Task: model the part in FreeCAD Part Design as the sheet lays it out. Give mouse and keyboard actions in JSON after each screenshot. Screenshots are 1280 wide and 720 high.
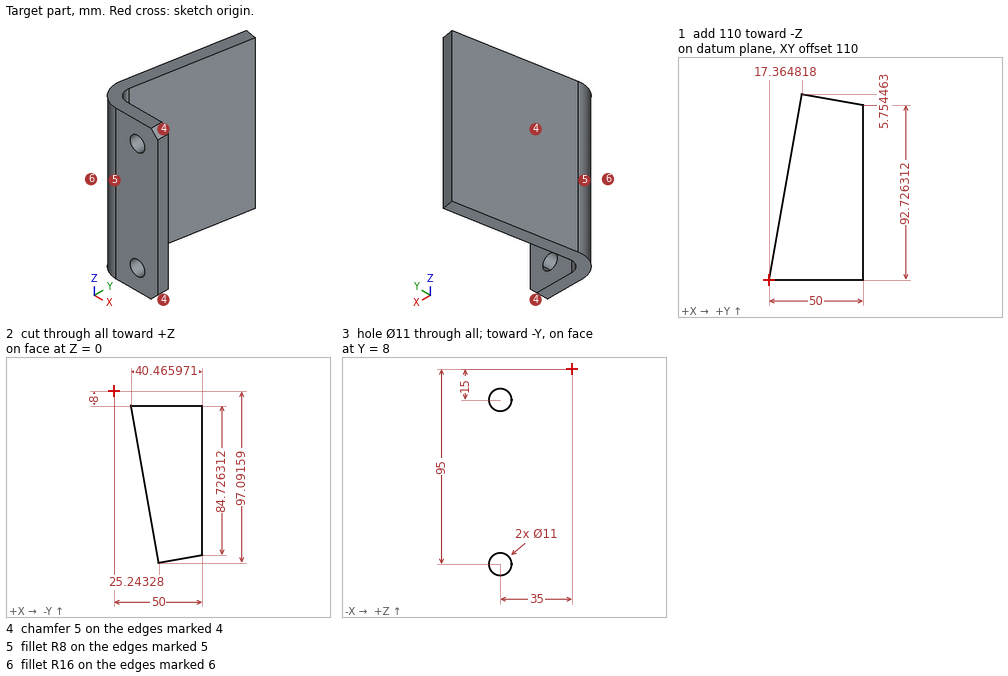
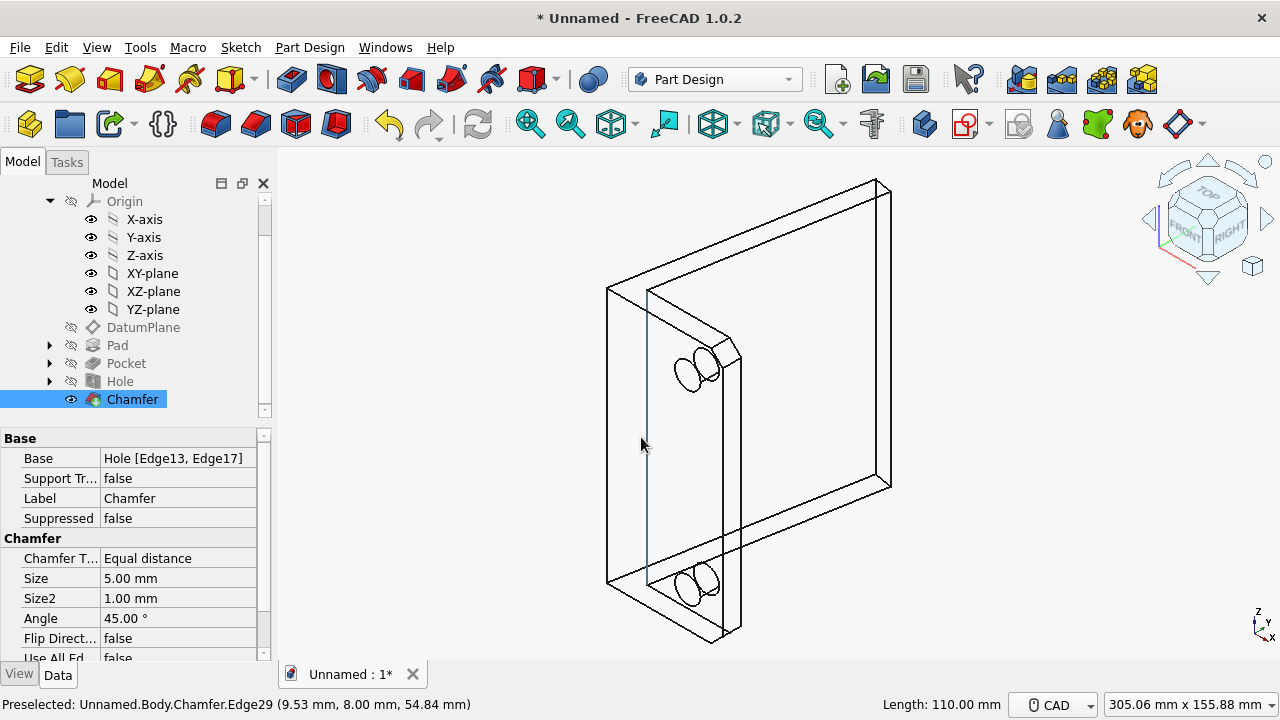
{"action": "key", "text": "v 1"}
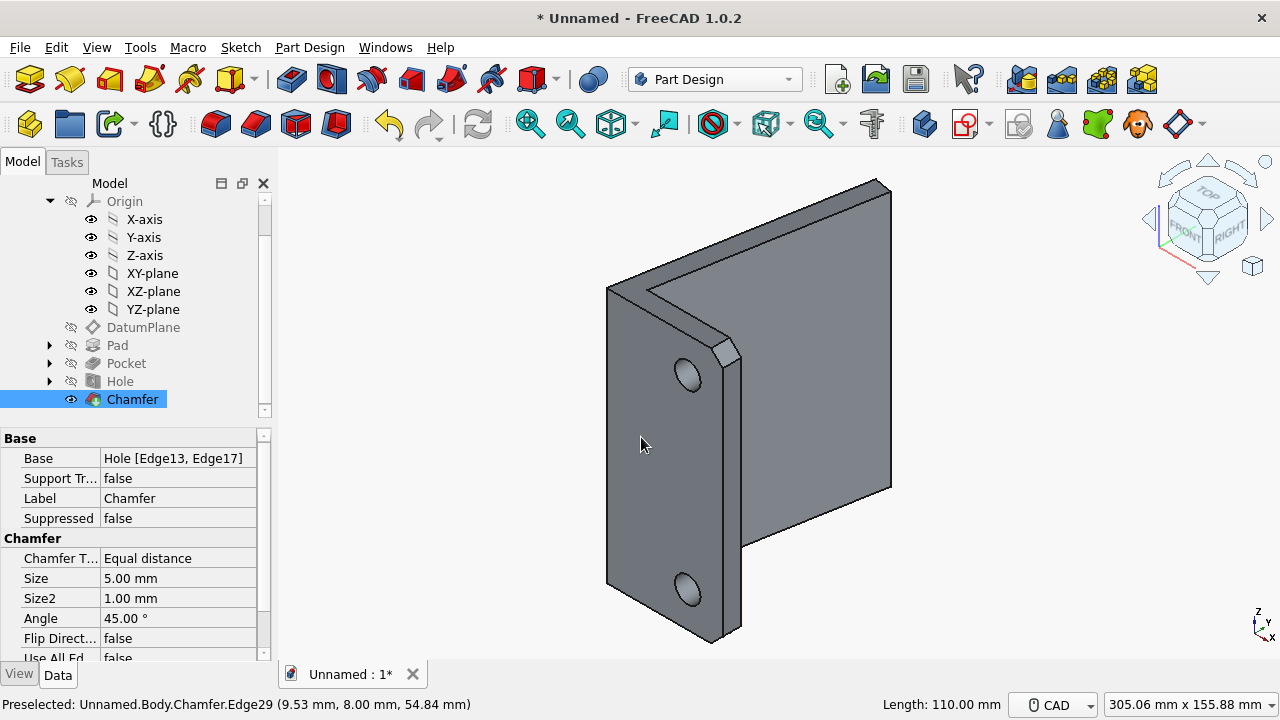
{"action": "left_click", "coordinate": [216, 124]}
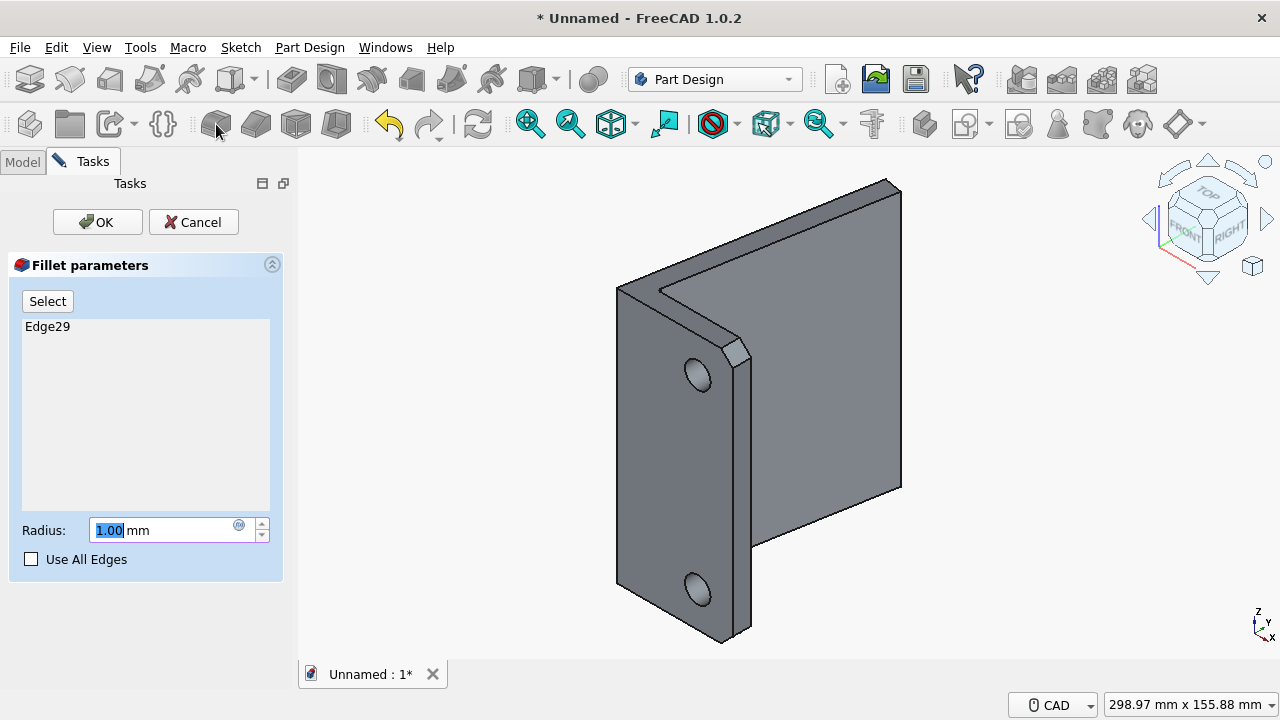
{"action": "type", "text": "8"}
{"action": "key", "text": "Tab"}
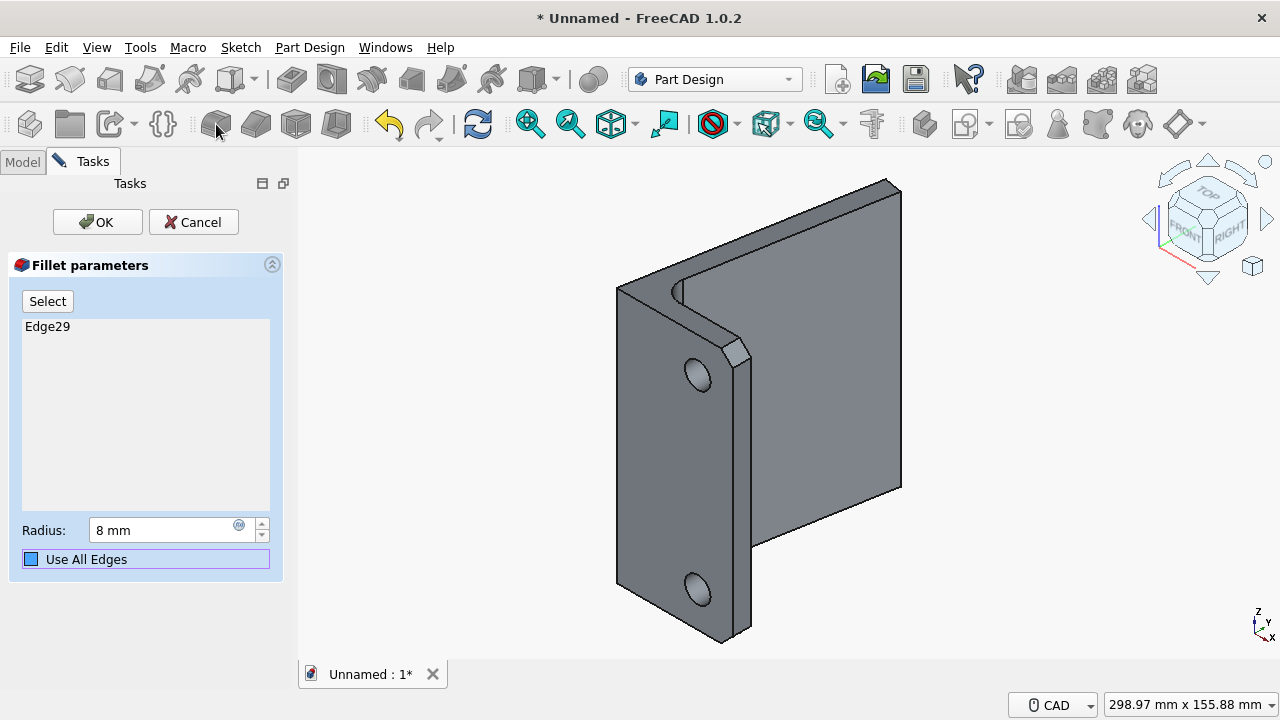
{"action": "left_click", "coordinate": [98, 222]}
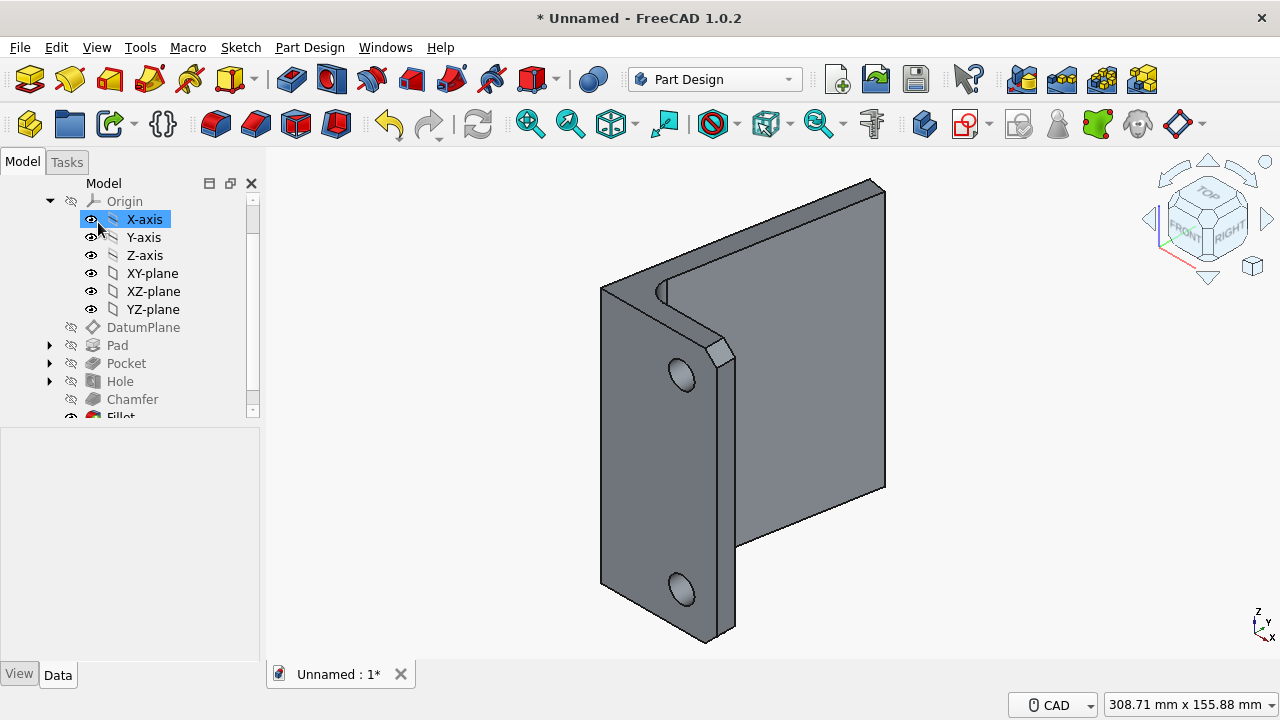
{"action": "key", "text": "2"}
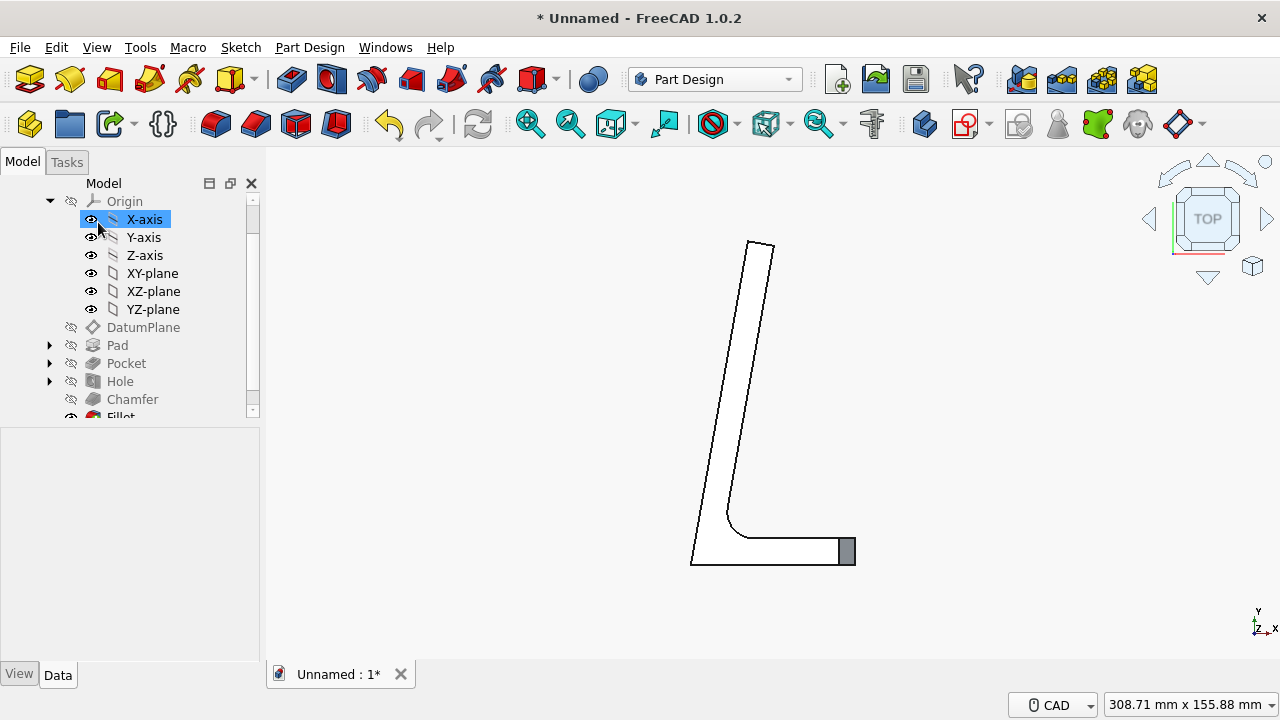
{"action": "key", "text": "0"}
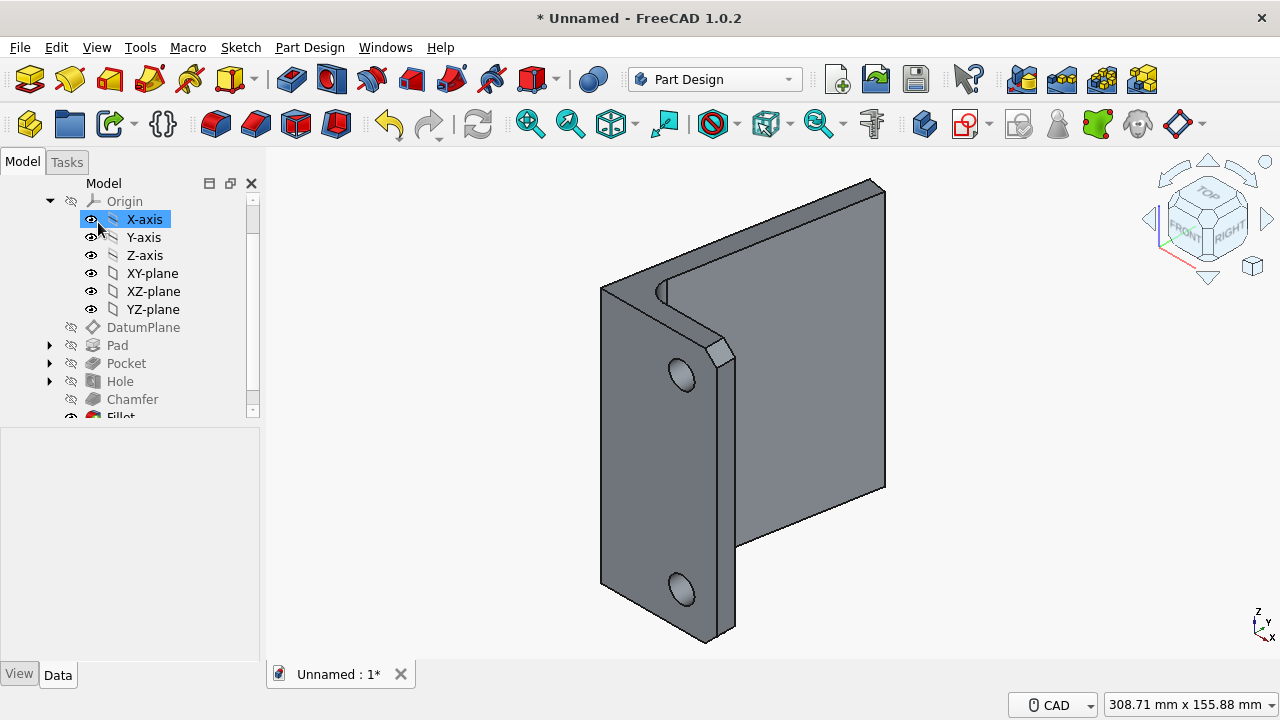
{"action": "key", "text": "1"}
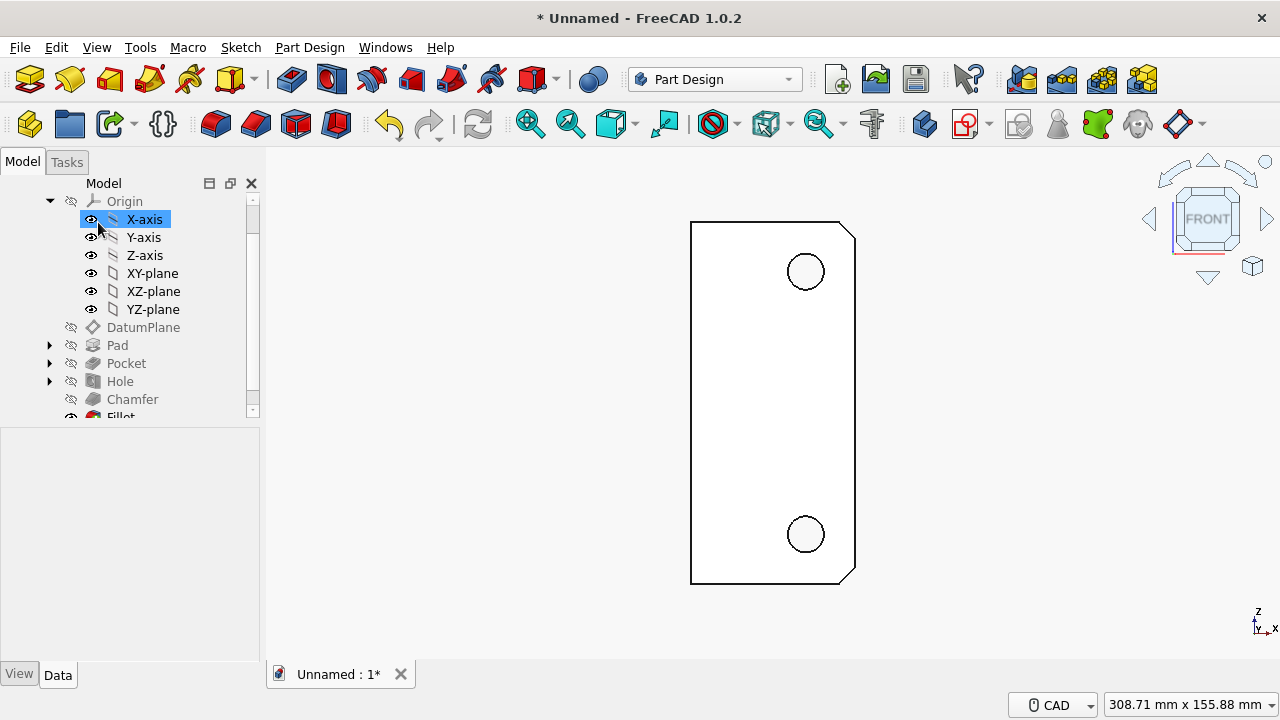
{"action": "key", "text": "3"}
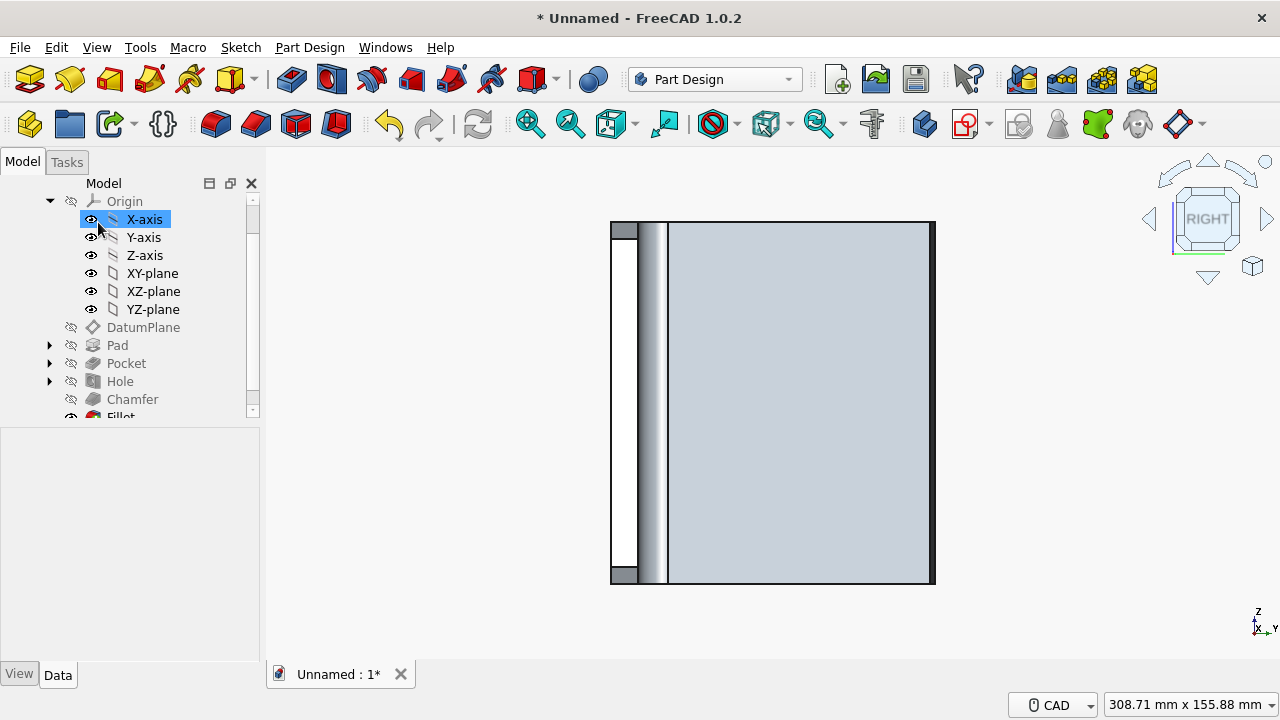
{"action": "key", "text": "5"}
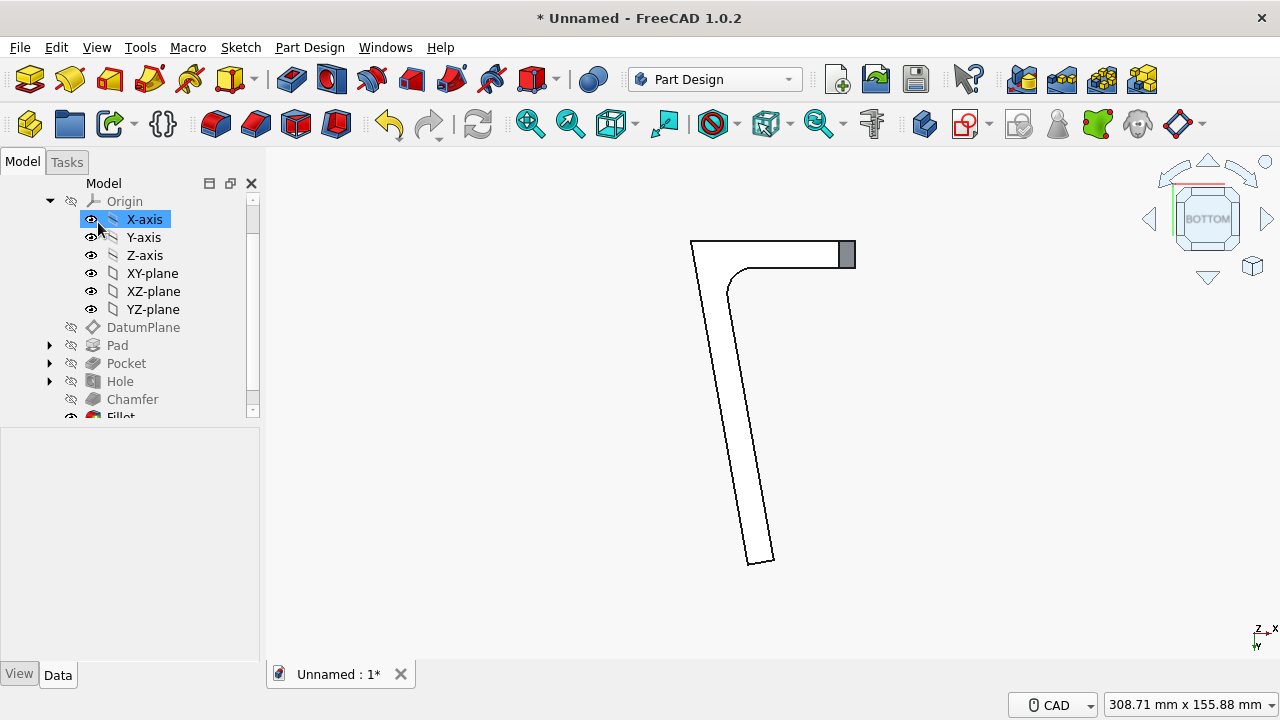
{"action": "key", "text": "4"}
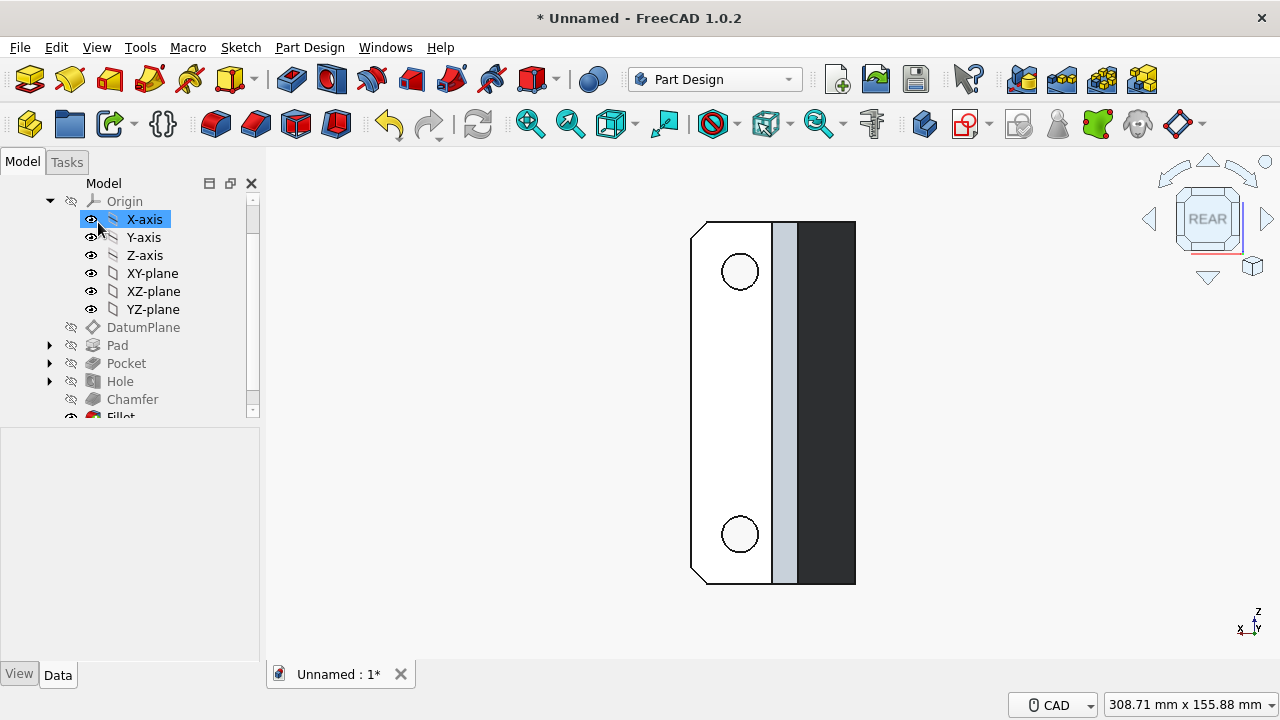
{"action": "key", "text": "6"}